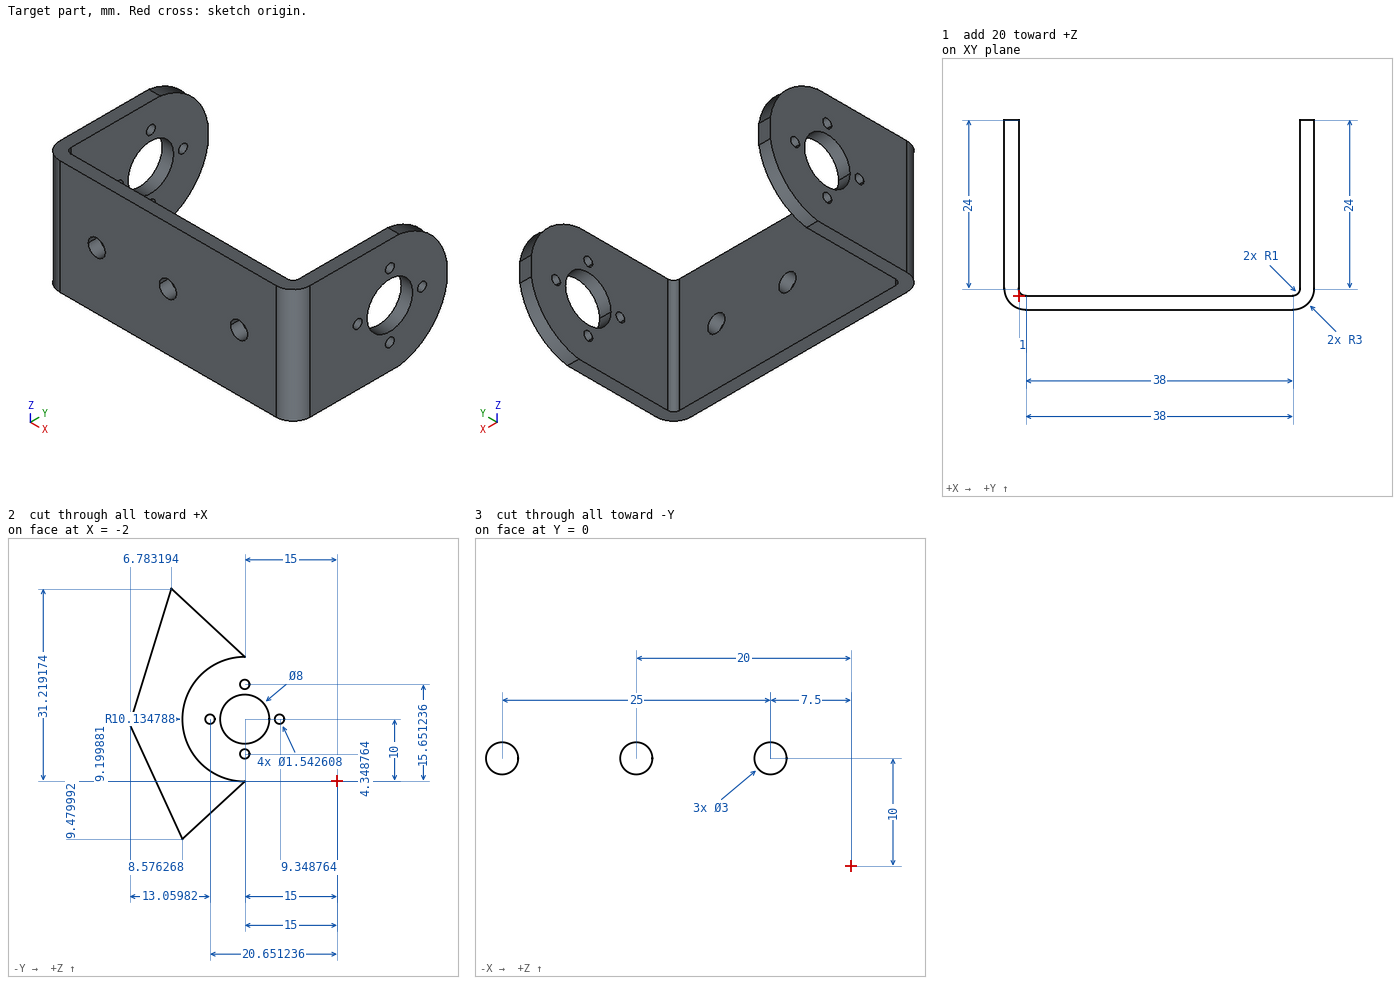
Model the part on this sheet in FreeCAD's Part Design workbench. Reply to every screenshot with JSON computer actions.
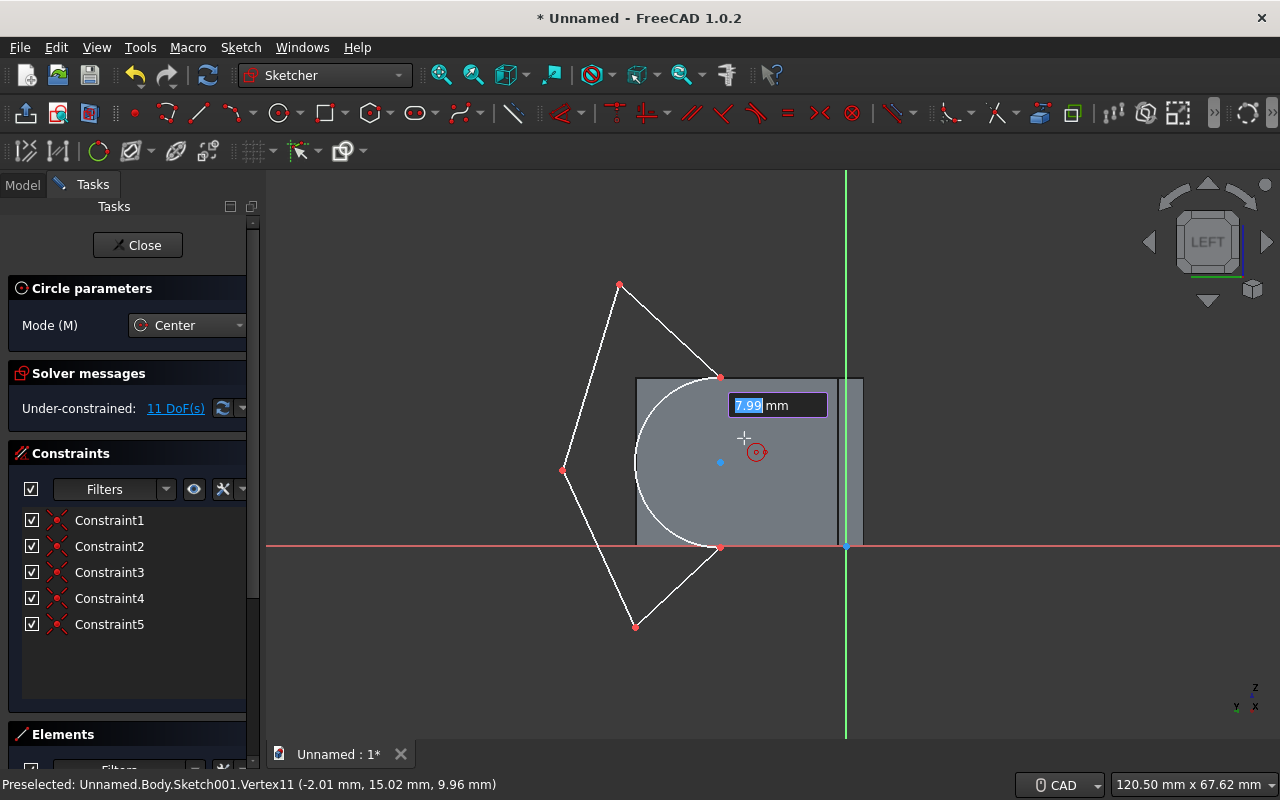
{"action": "type", "text": "8"}
{"action": "key", "text": "Return"}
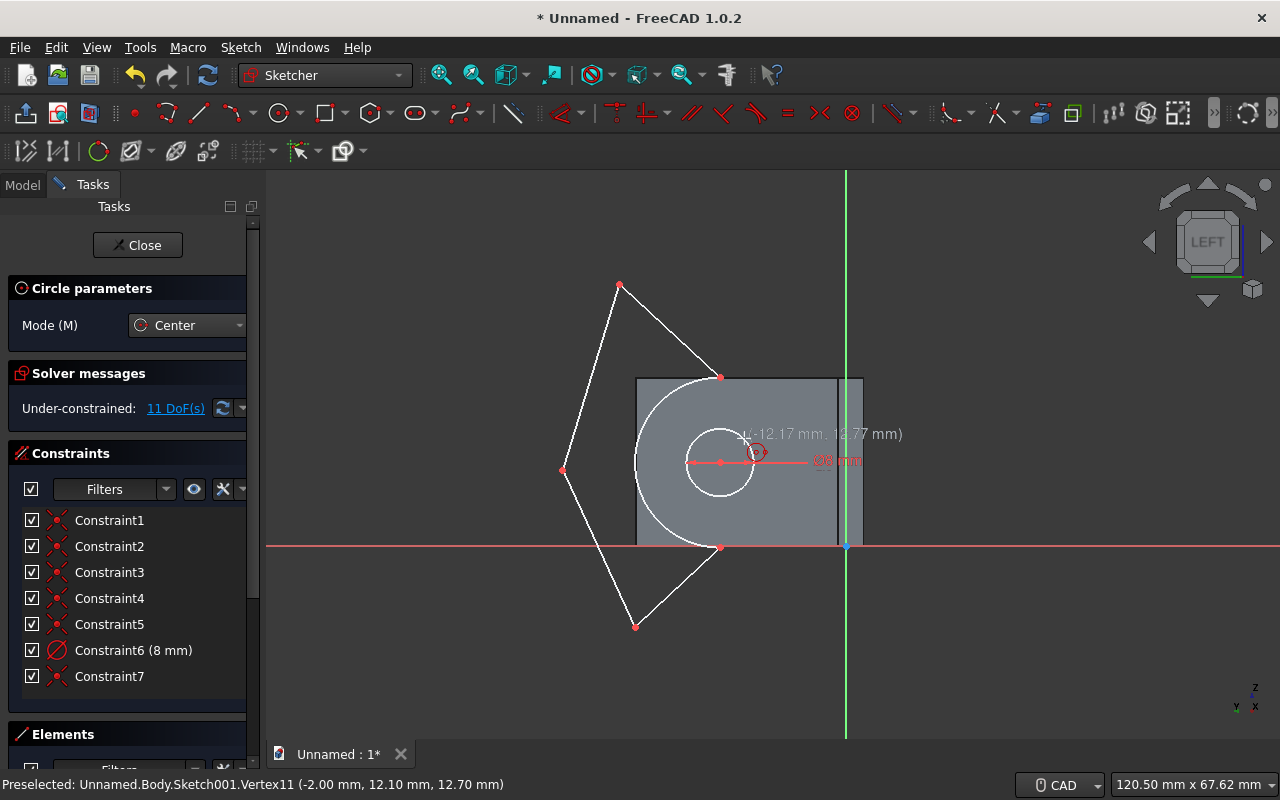
{"action": "scroll", "coordinate": [673, 462], "scroll_direction": "up", "scroll_amount": 7}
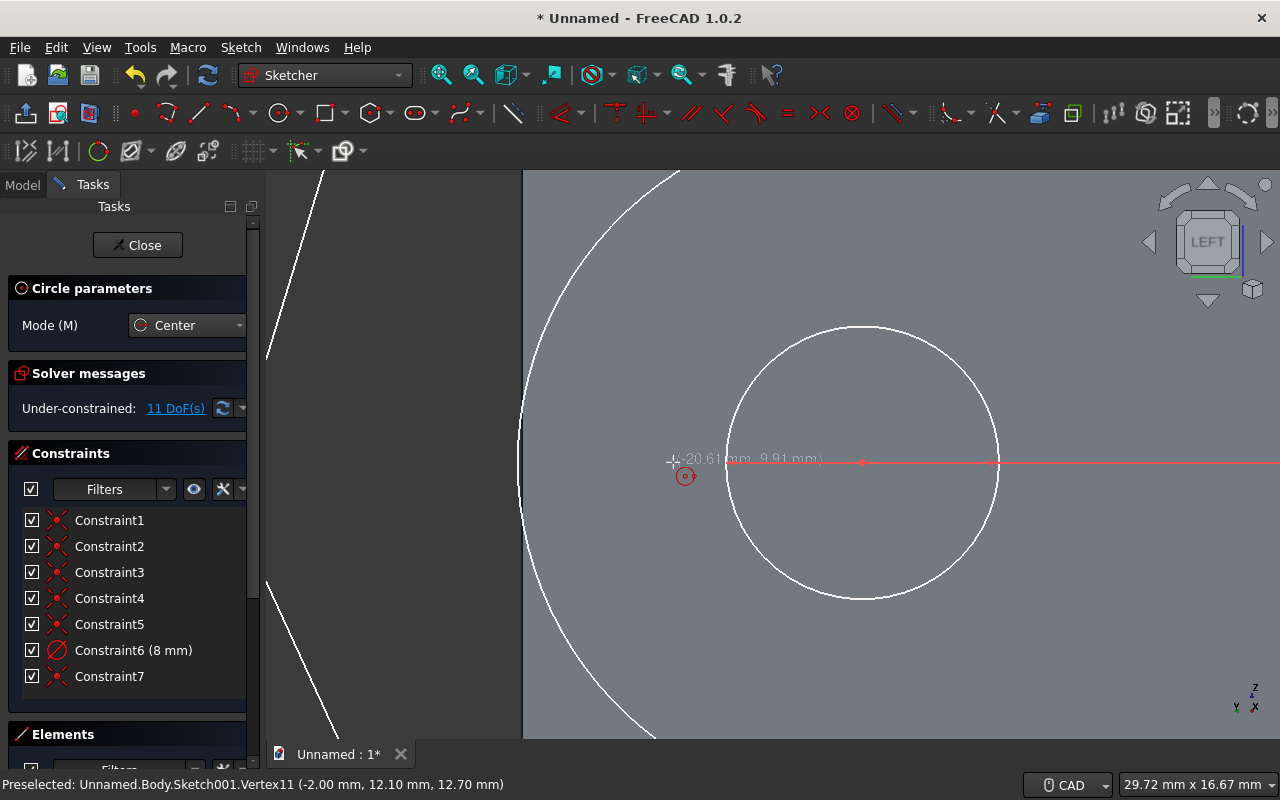
{"action": "left_click", "coordinate": [670, 462]}
{"action": "mouse_move", "coordinate": [689, 443]}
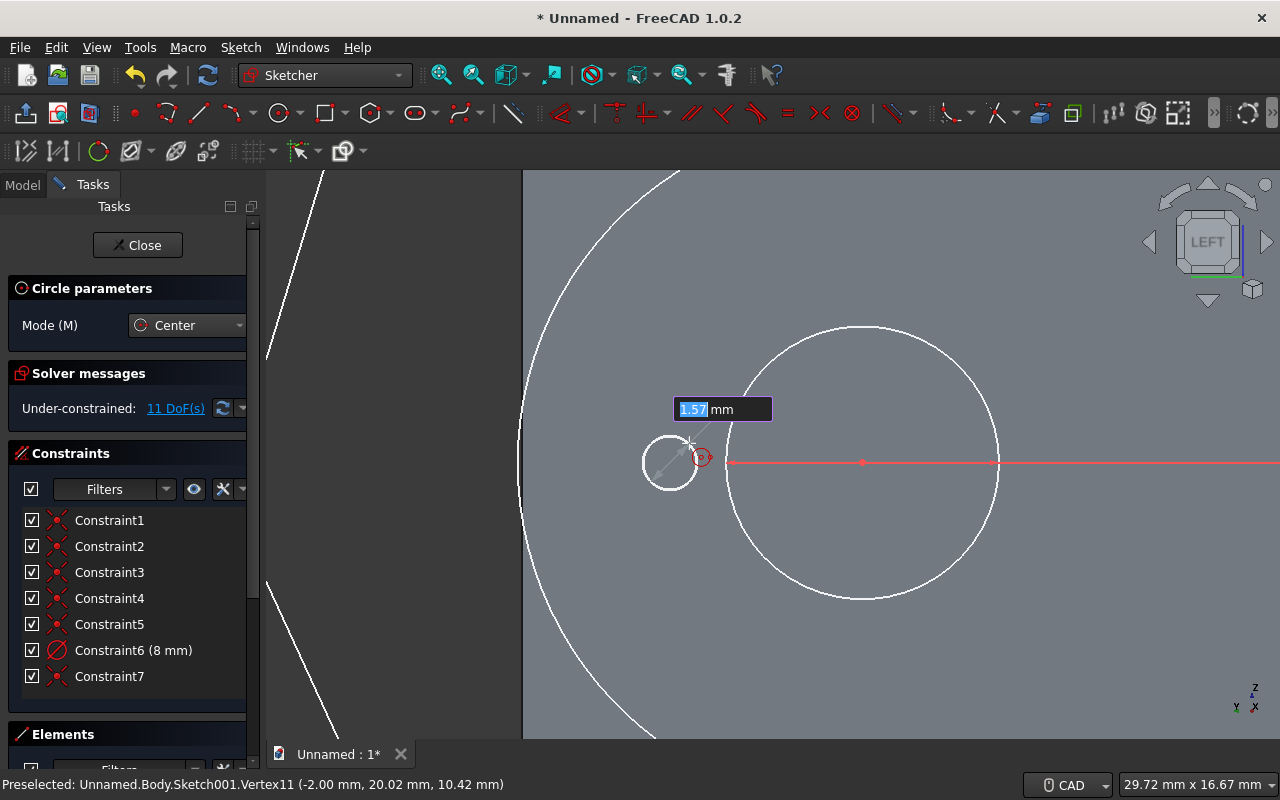
{"action": "type", "text": "1.542608"}
{"action": "key", "text": "Return"}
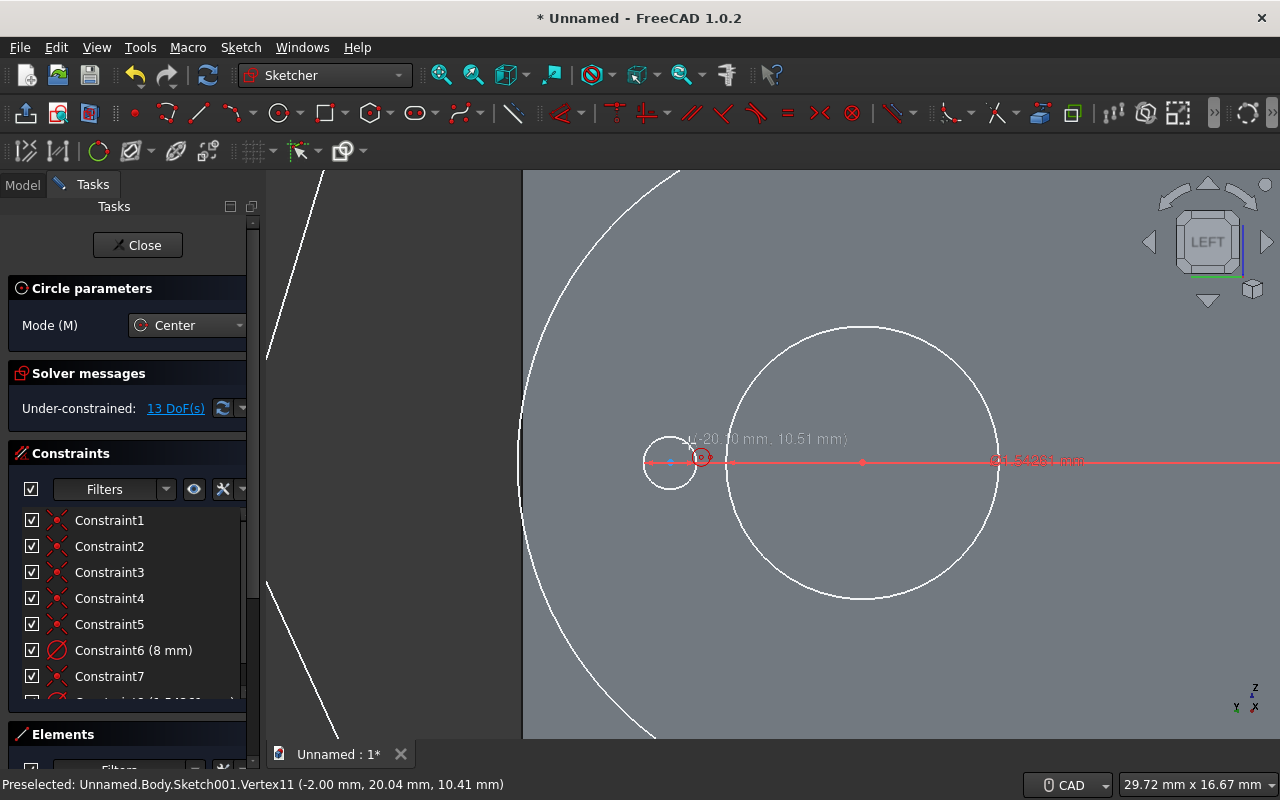
{"action": "left_click", "coordinate": [863, 269]}
{"action": "mouse_move", "coordinate": [882, 250]}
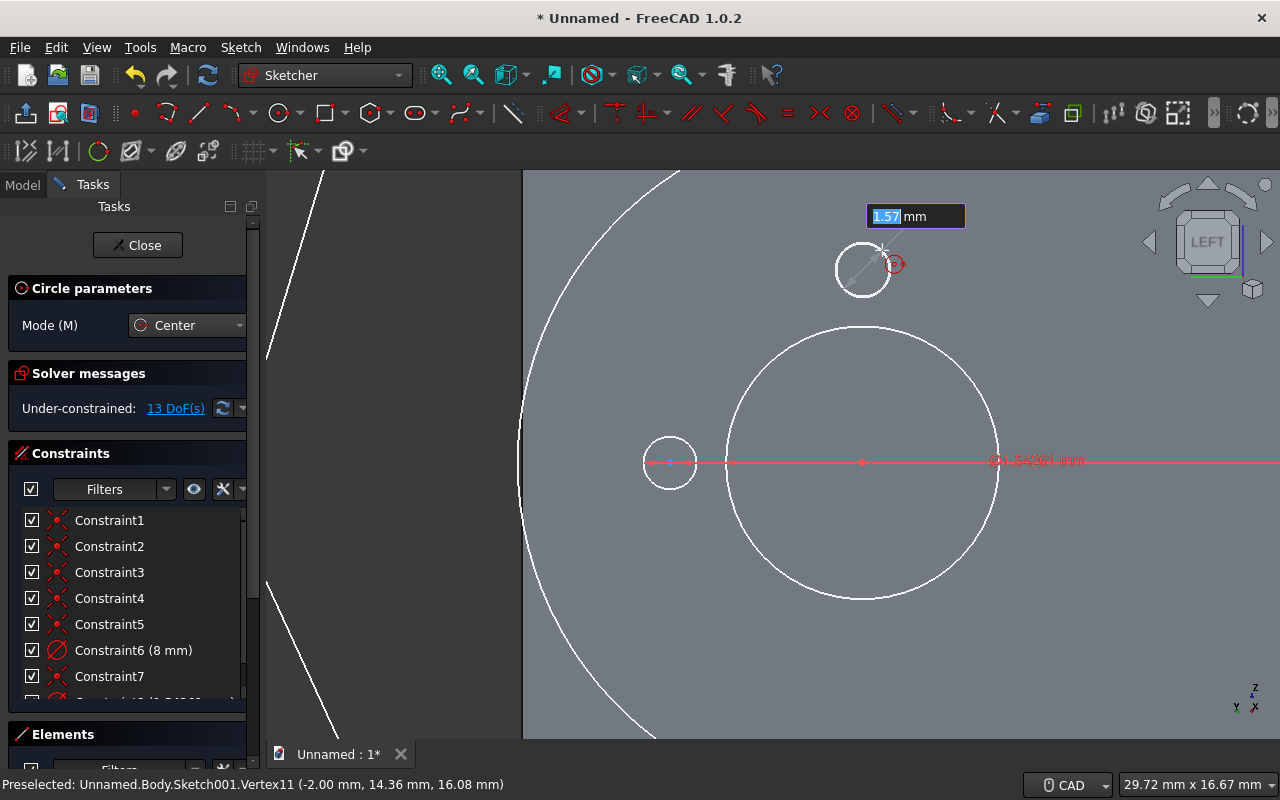
{"action": "type", "text": "1.542608"}
{"action": "key", "text": "Return"}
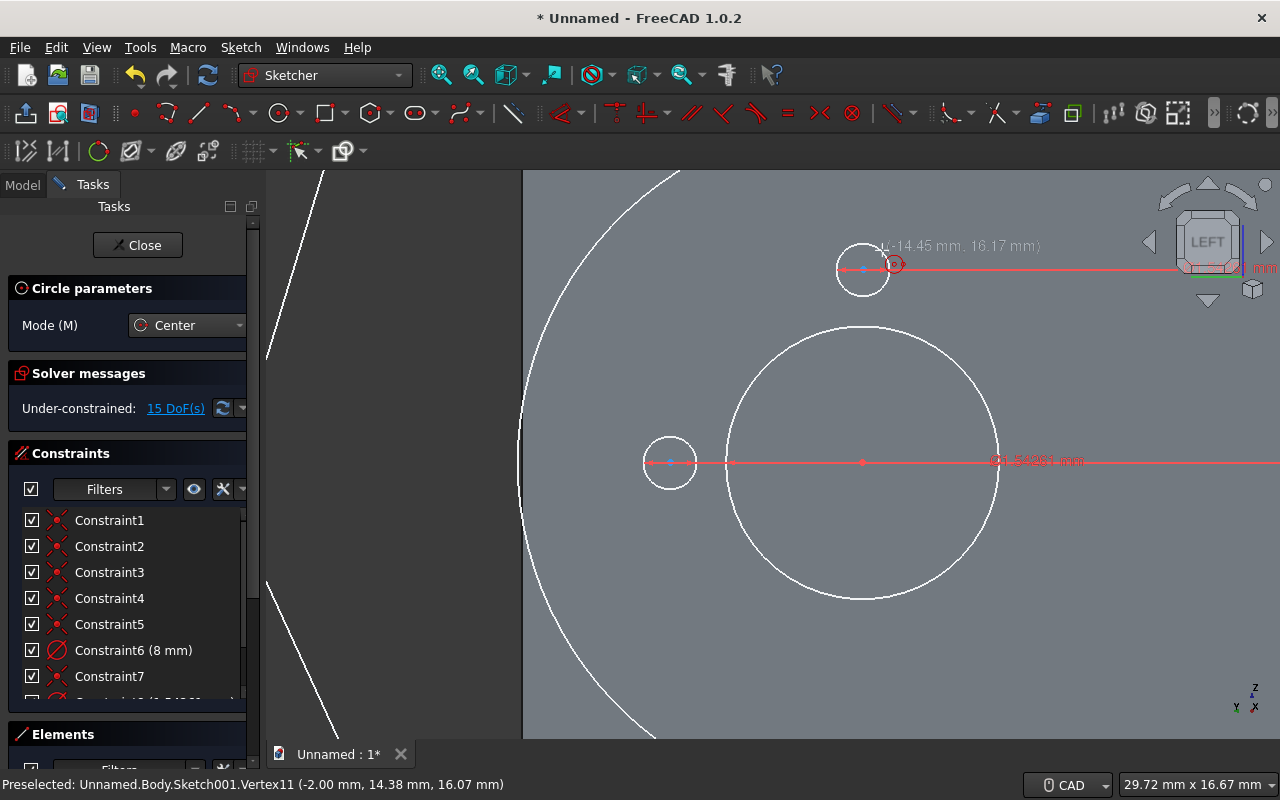
{"action": "left_click", "coordinate": [1056, 462]}
{"action": "mouse_move", "coordinate": [1075, 443]}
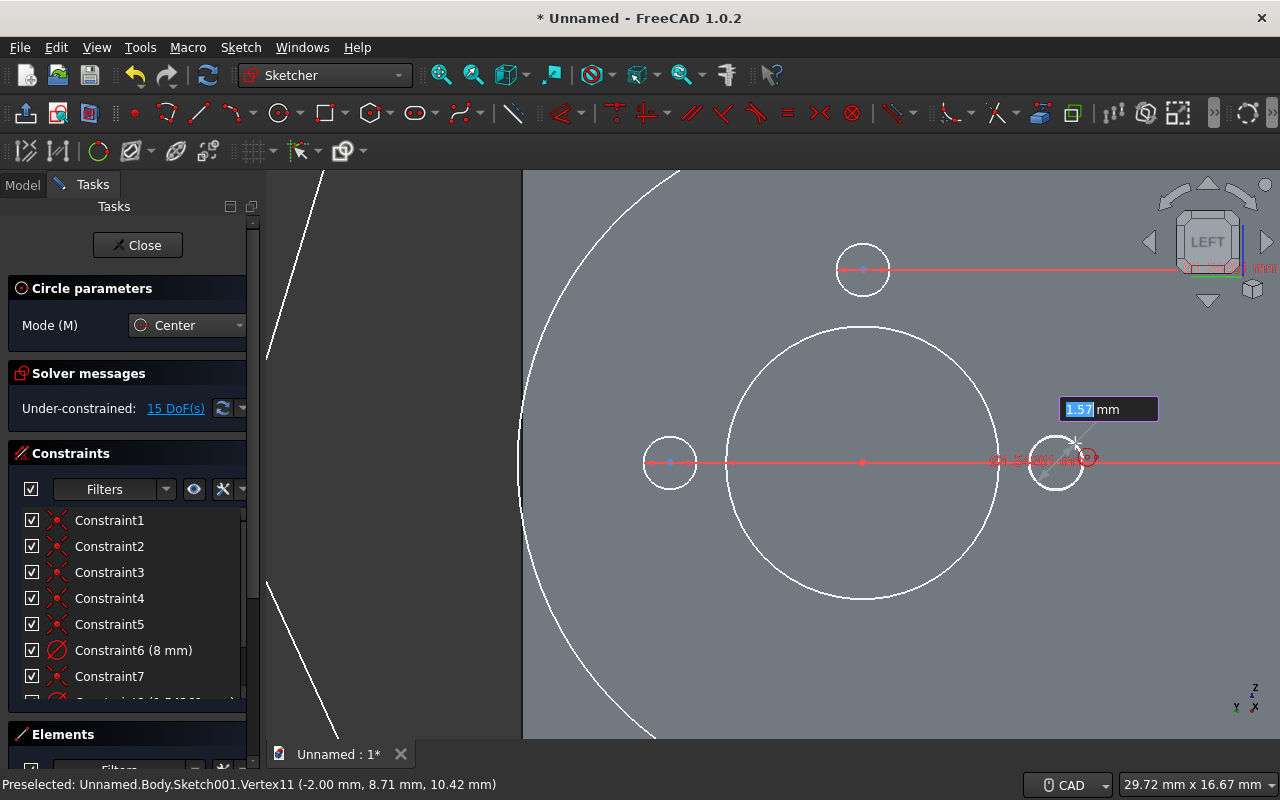
{"action": "type", "text": "1.542608"}
{"action": "key", "text": "Return"}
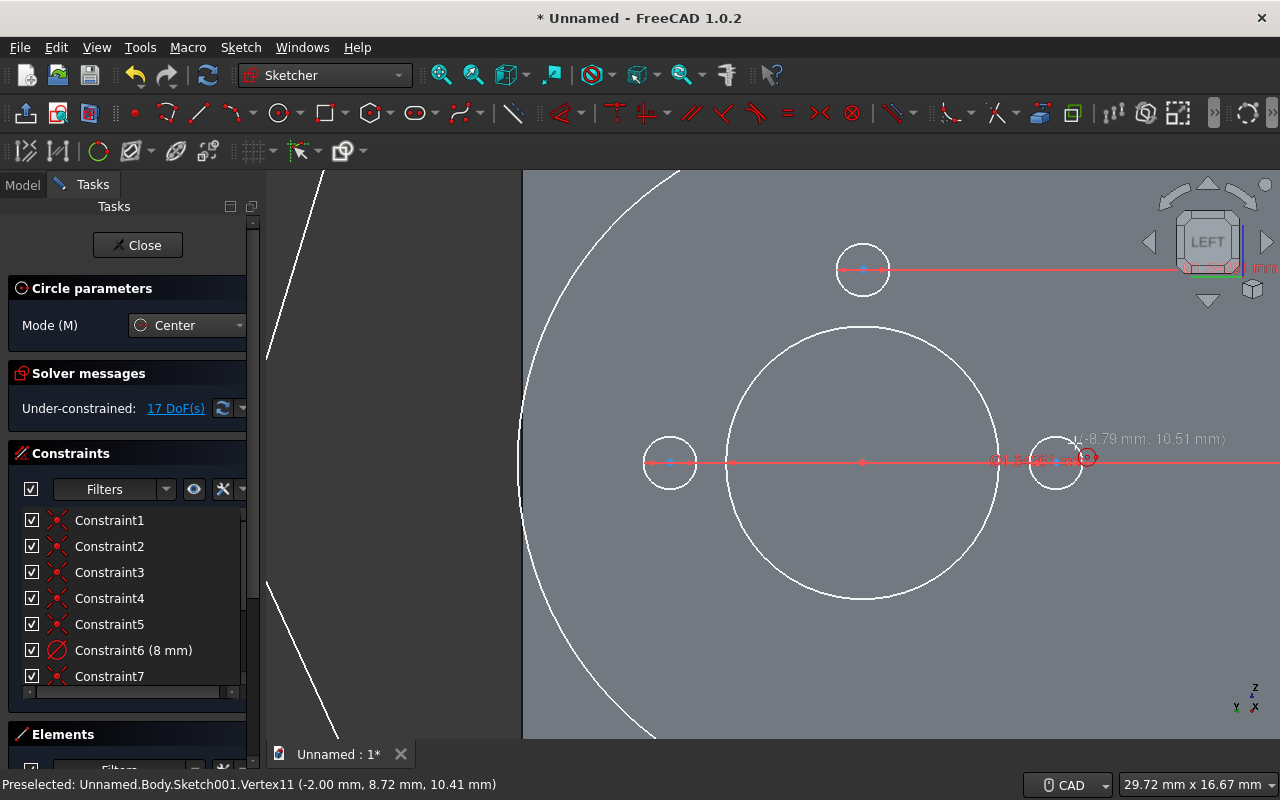
{"action": "left_click", "coordinate": [863, 654]}
{"action": "mouse_move", "coordinate": [882, 636]}